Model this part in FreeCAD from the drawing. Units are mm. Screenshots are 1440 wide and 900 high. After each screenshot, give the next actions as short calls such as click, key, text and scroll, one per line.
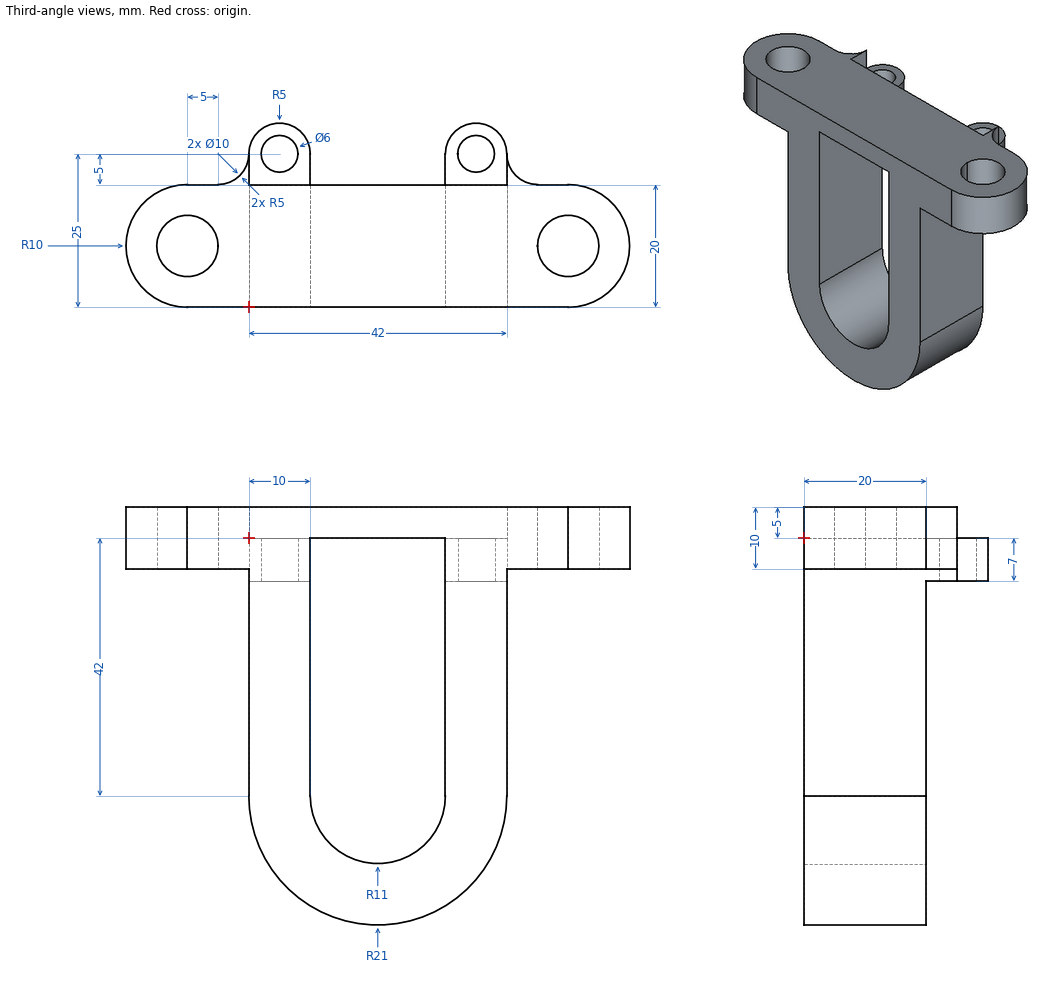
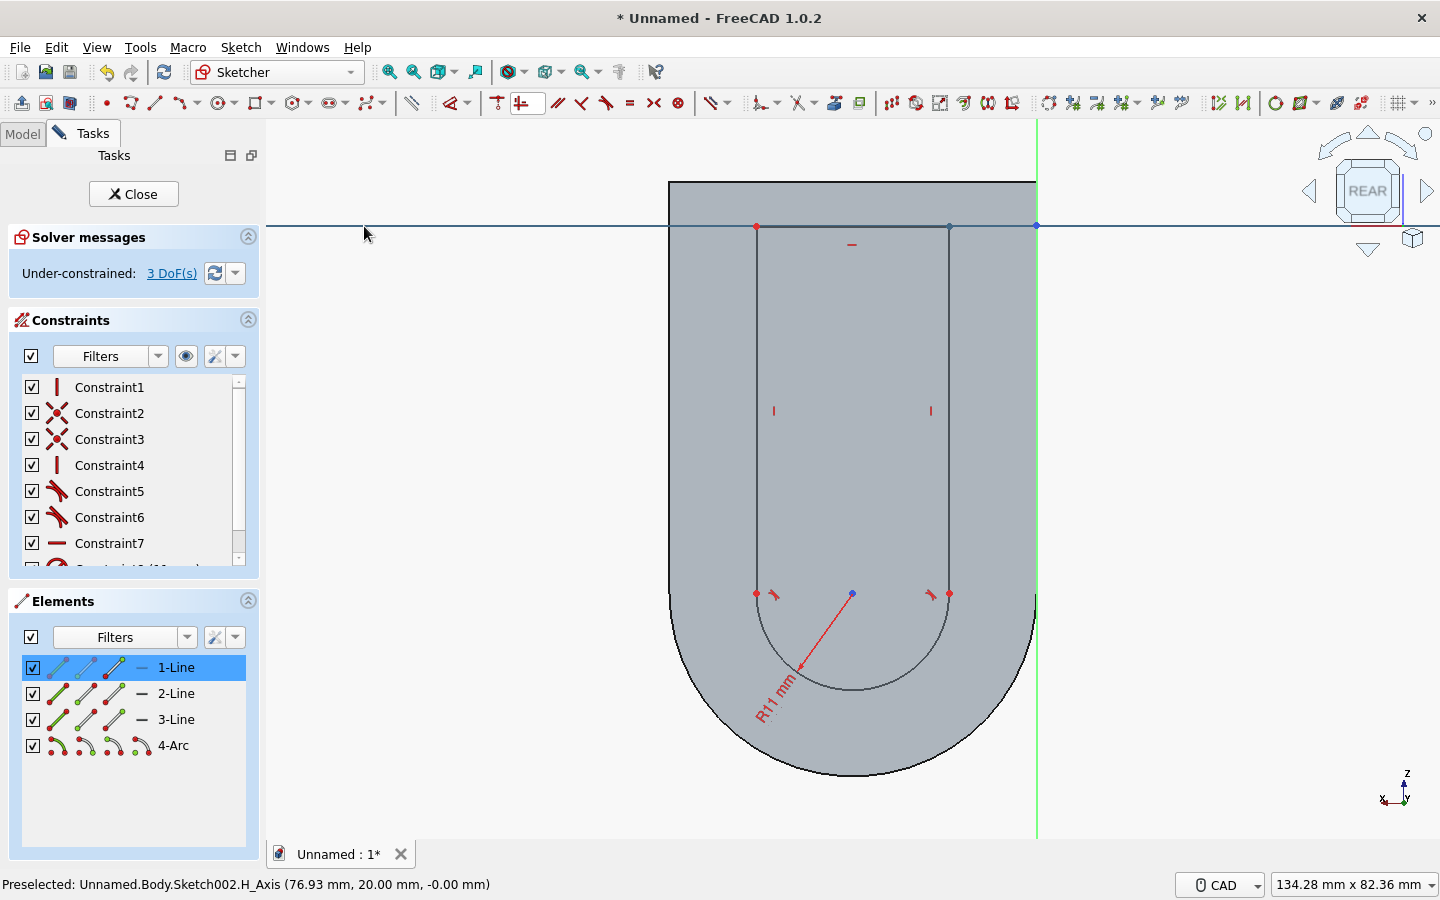
click(498, 104)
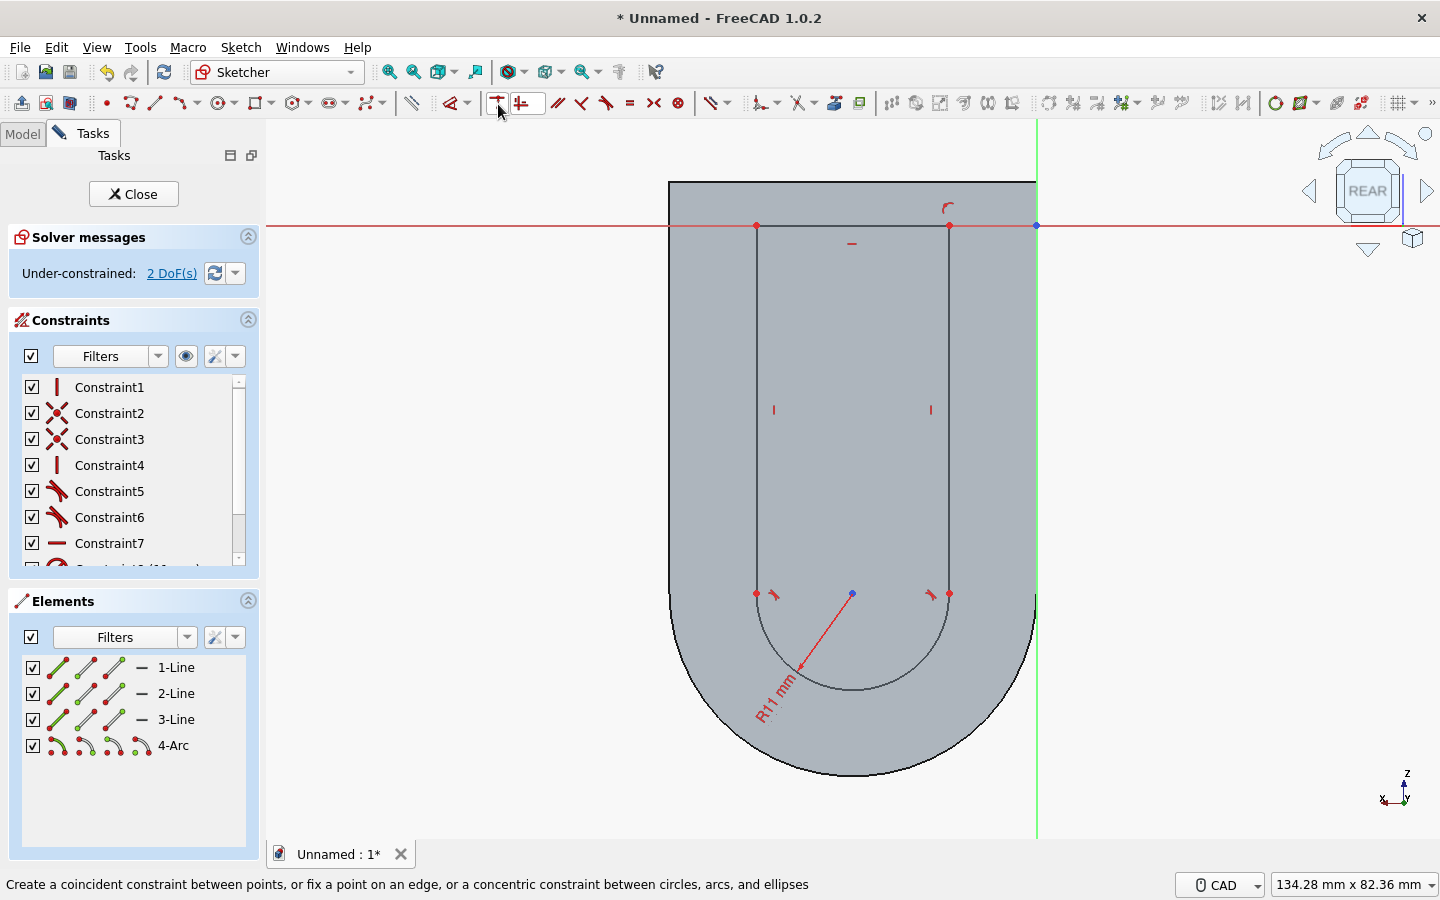
click(450, 104)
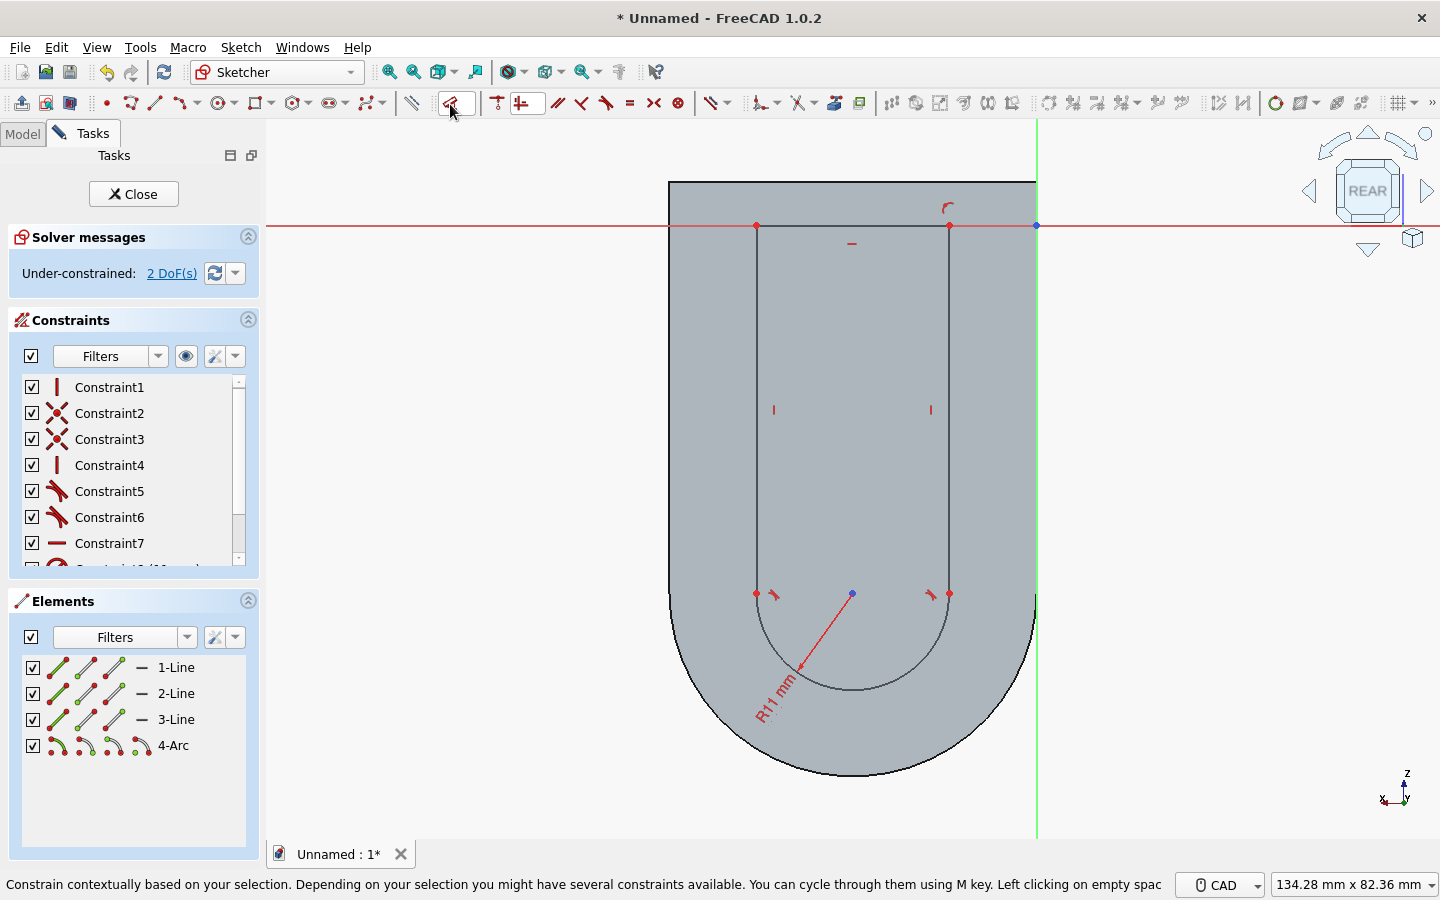
click(949, 483)
click(983, 410)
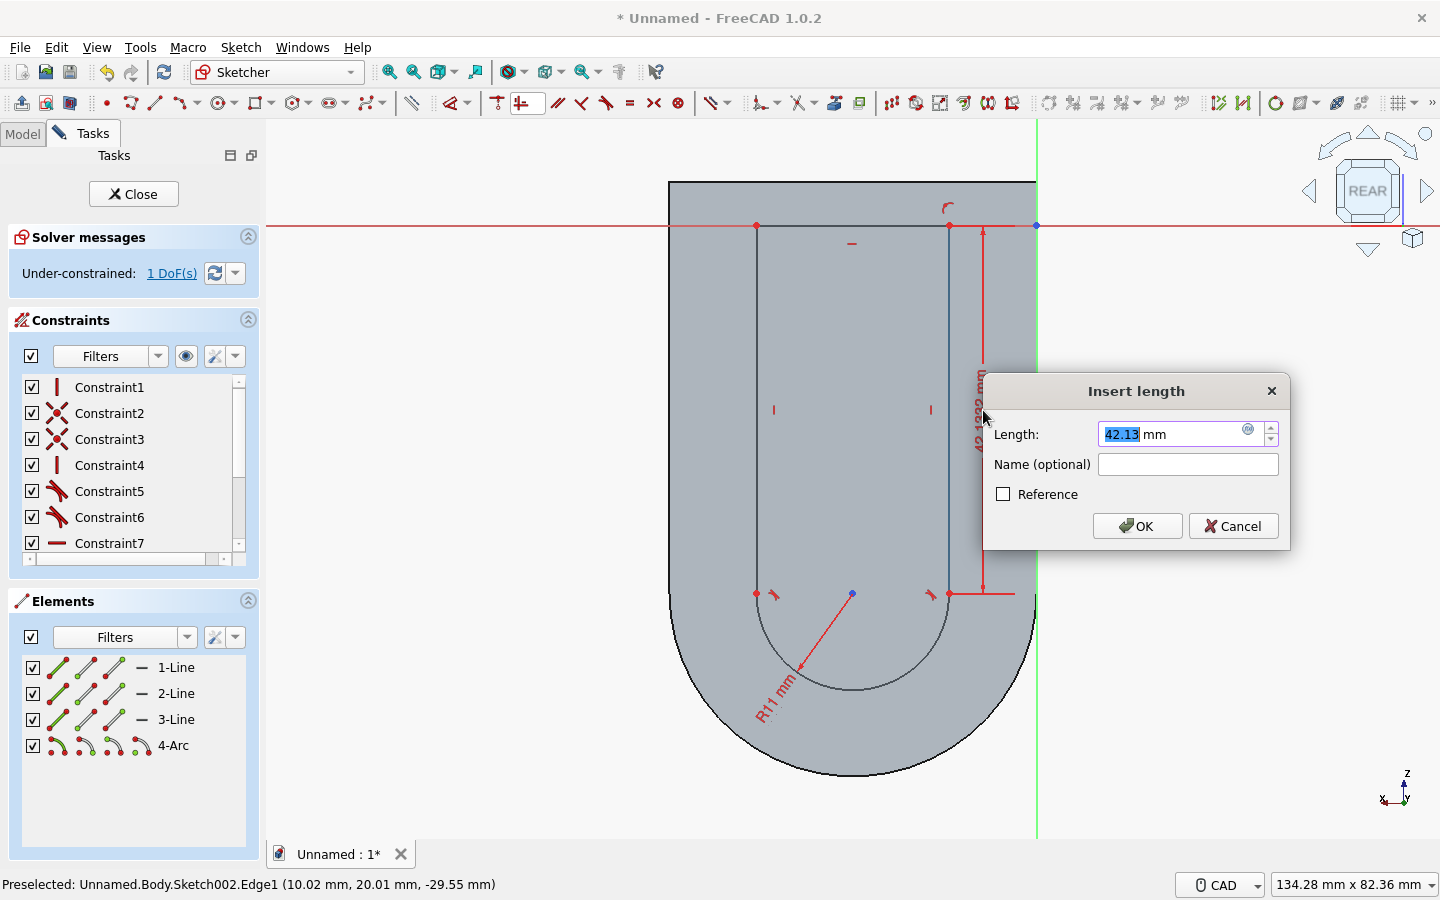
text(42)
key(Return)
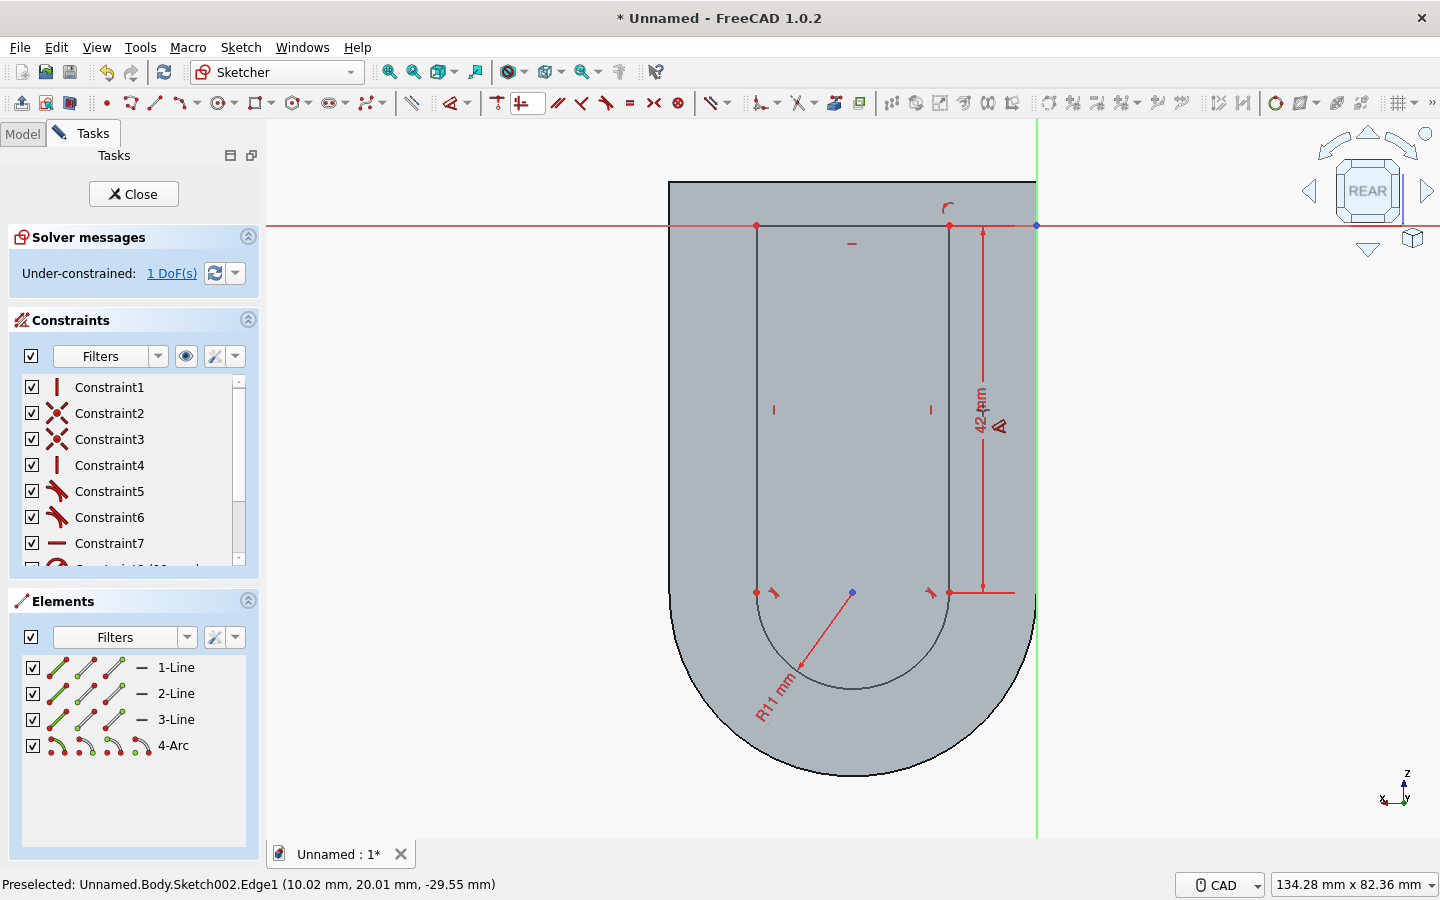
click(949, 593)
click(993, 192)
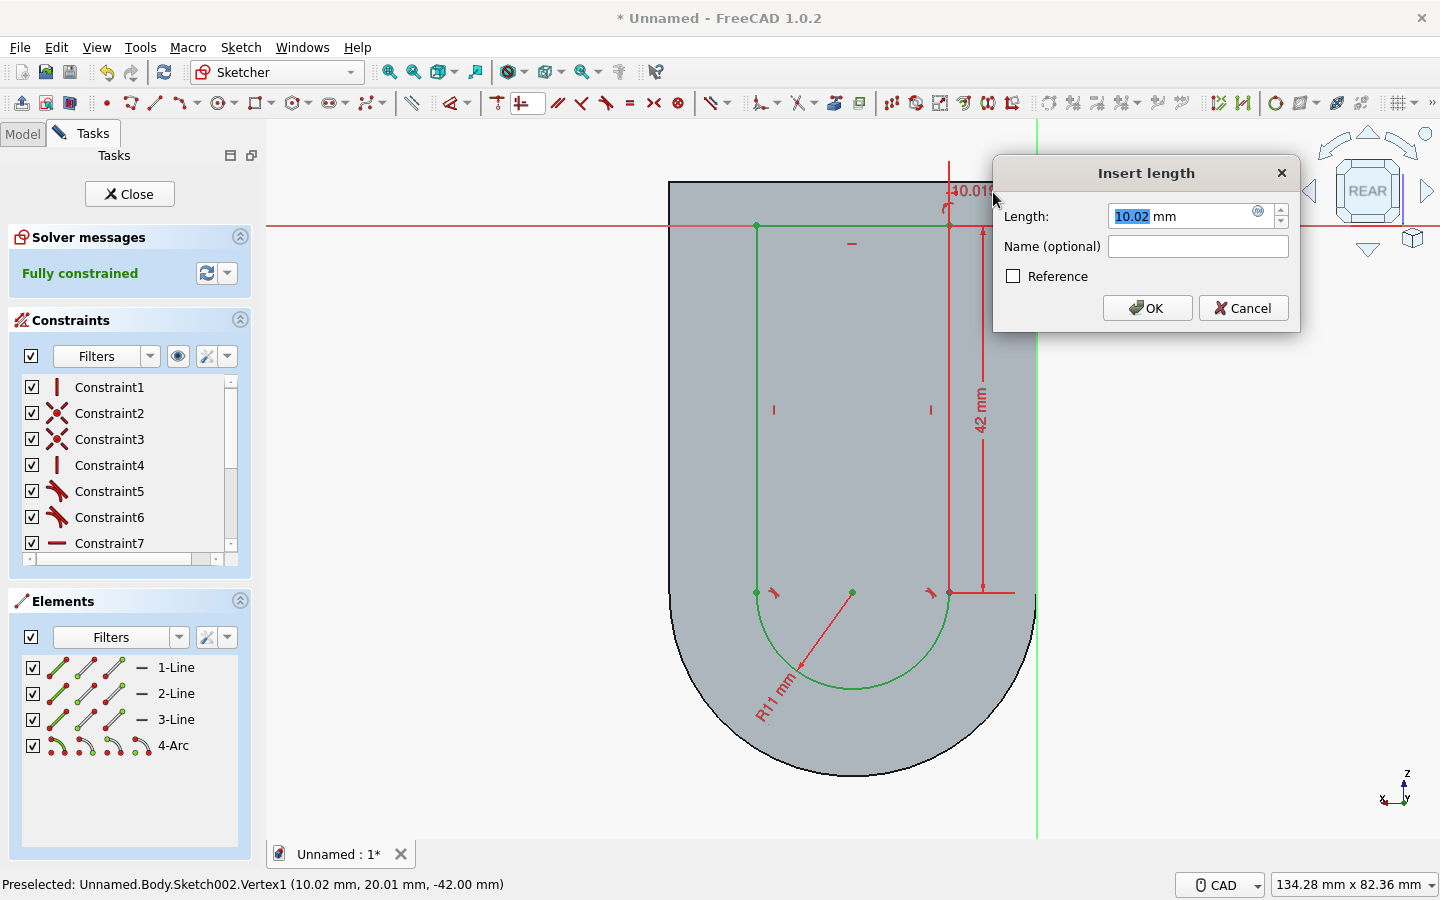
text(10)
key(Return)
key(Escape)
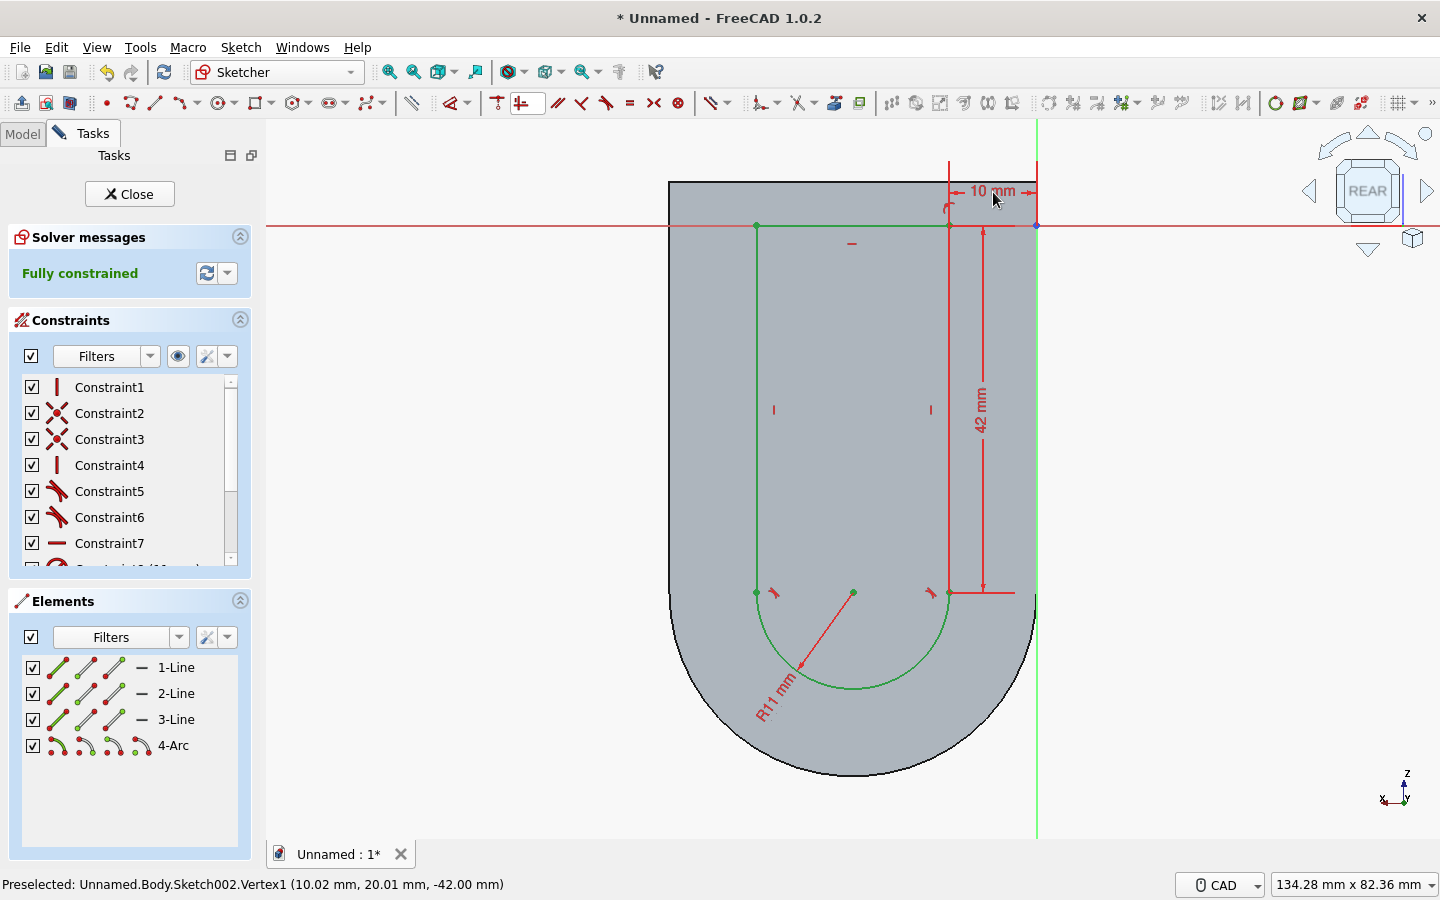
click(130, 194)